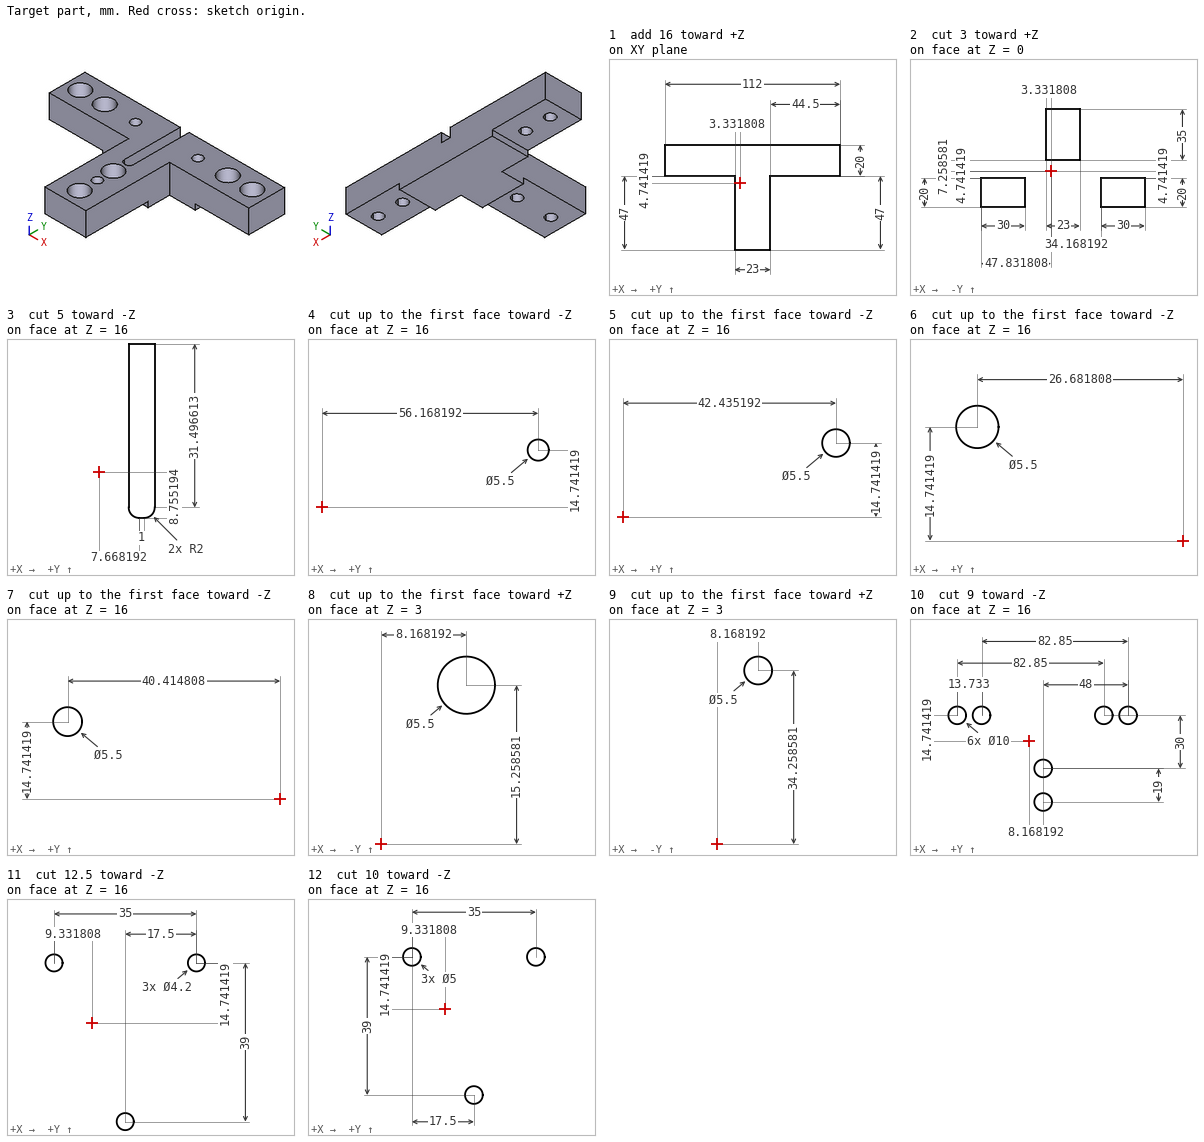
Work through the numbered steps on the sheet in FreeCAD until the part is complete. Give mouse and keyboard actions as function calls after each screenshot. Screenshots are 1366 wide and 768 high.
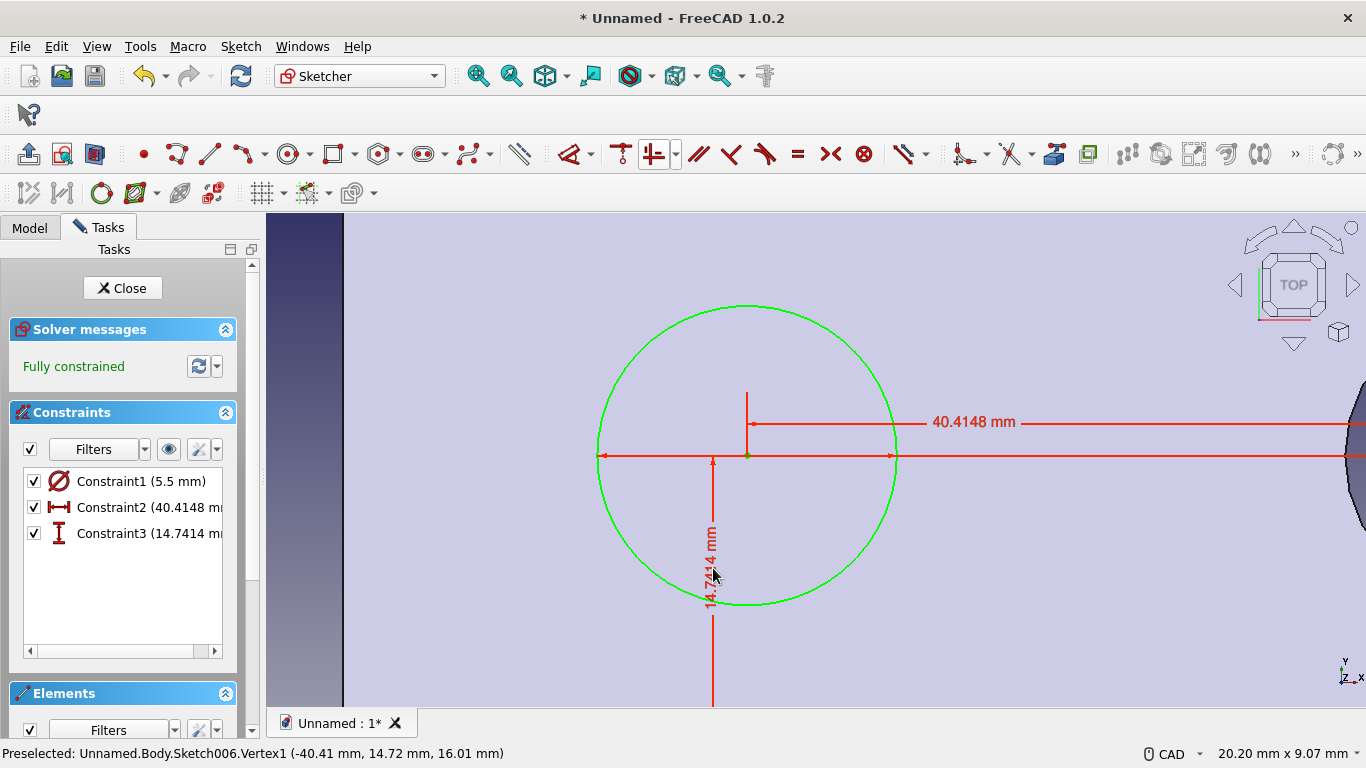
click(123, 288)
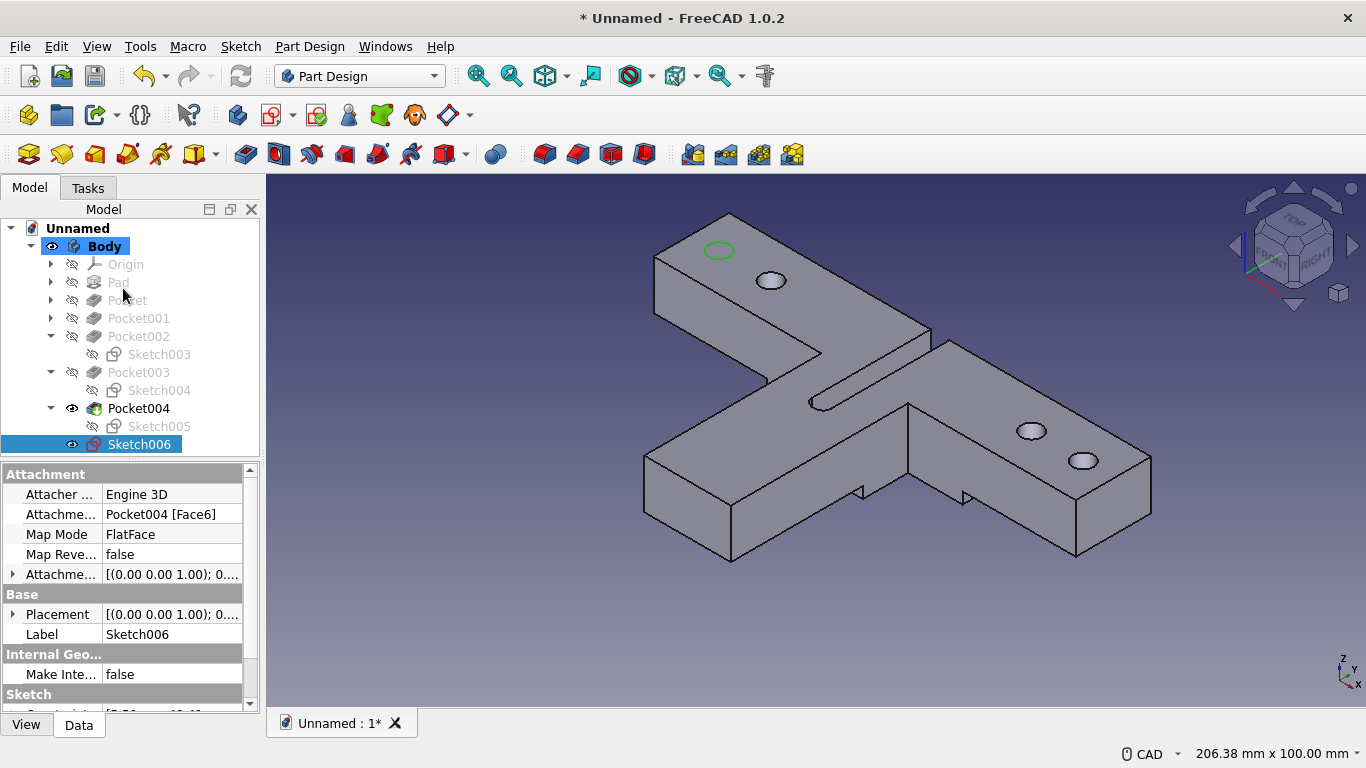
click(246, 154)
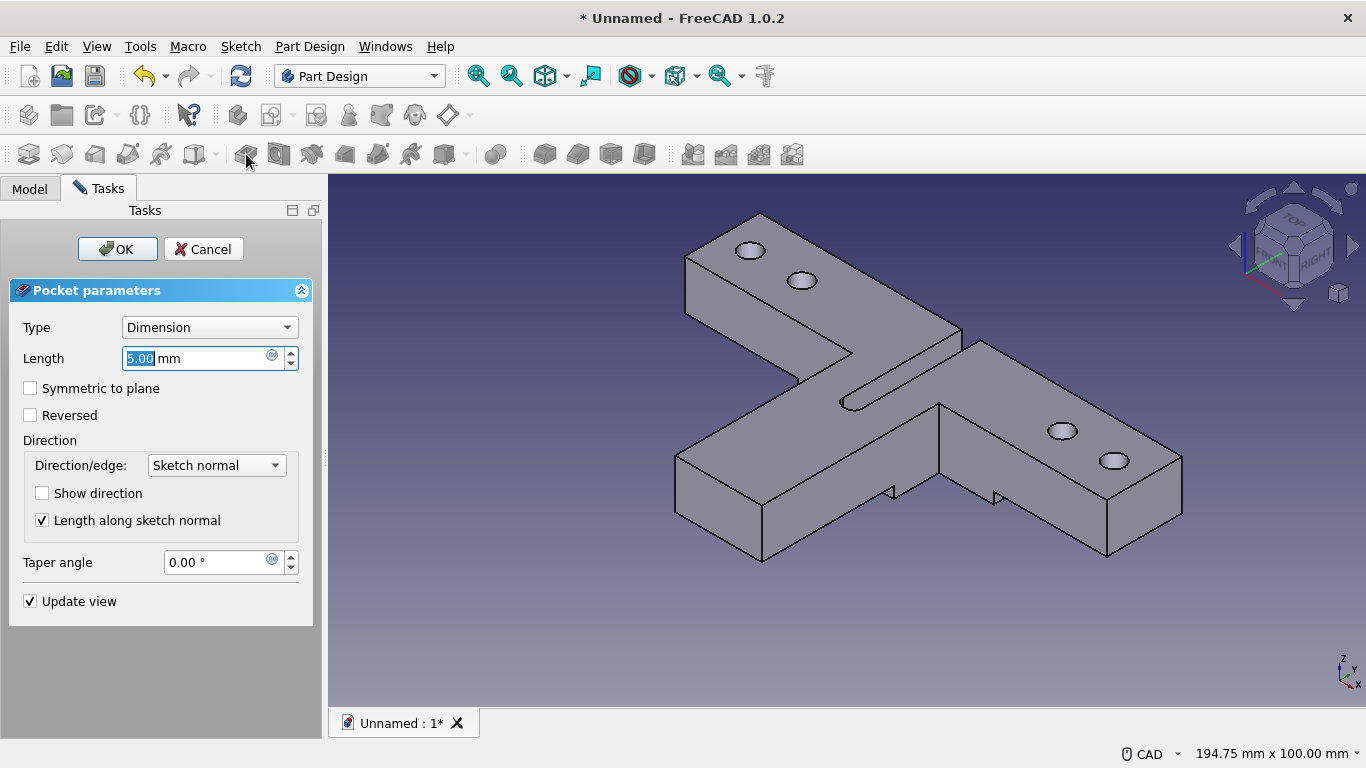
click(210, 328)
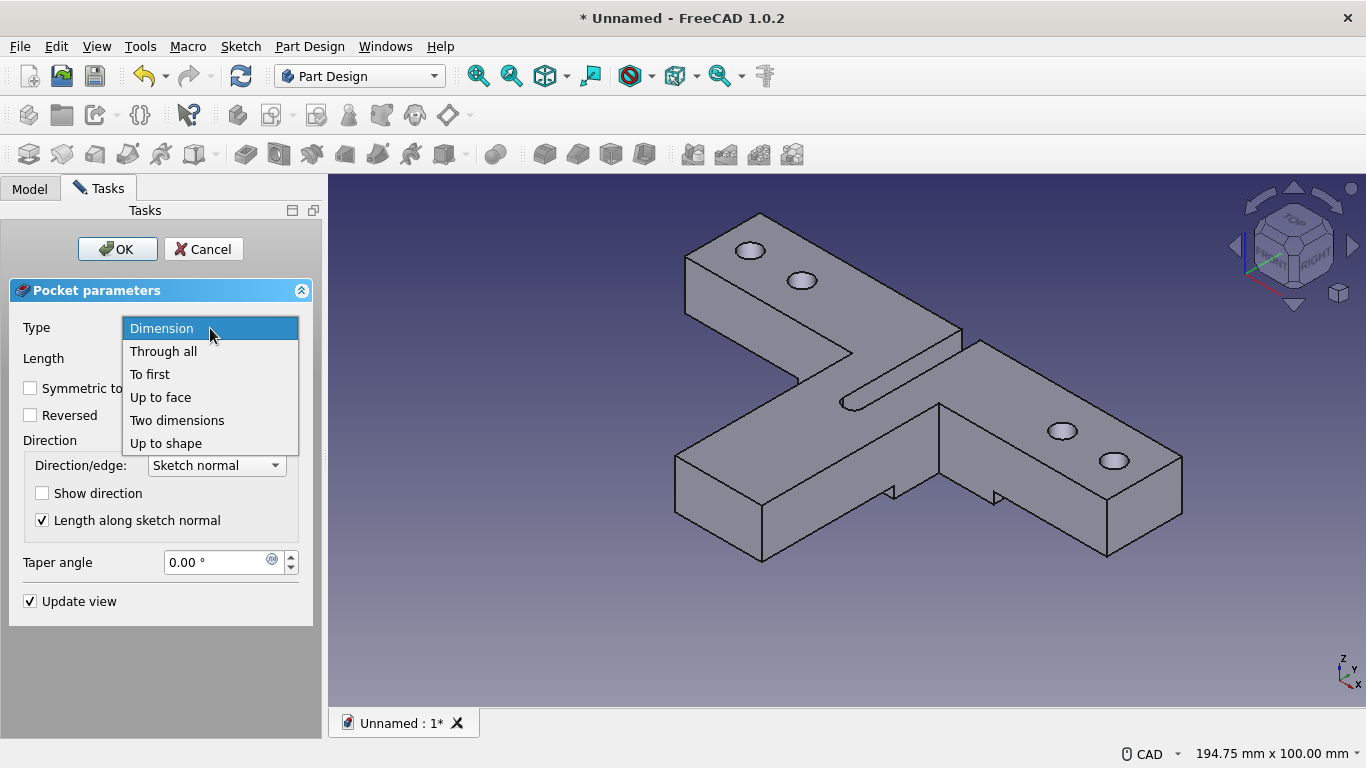
click(208, 374)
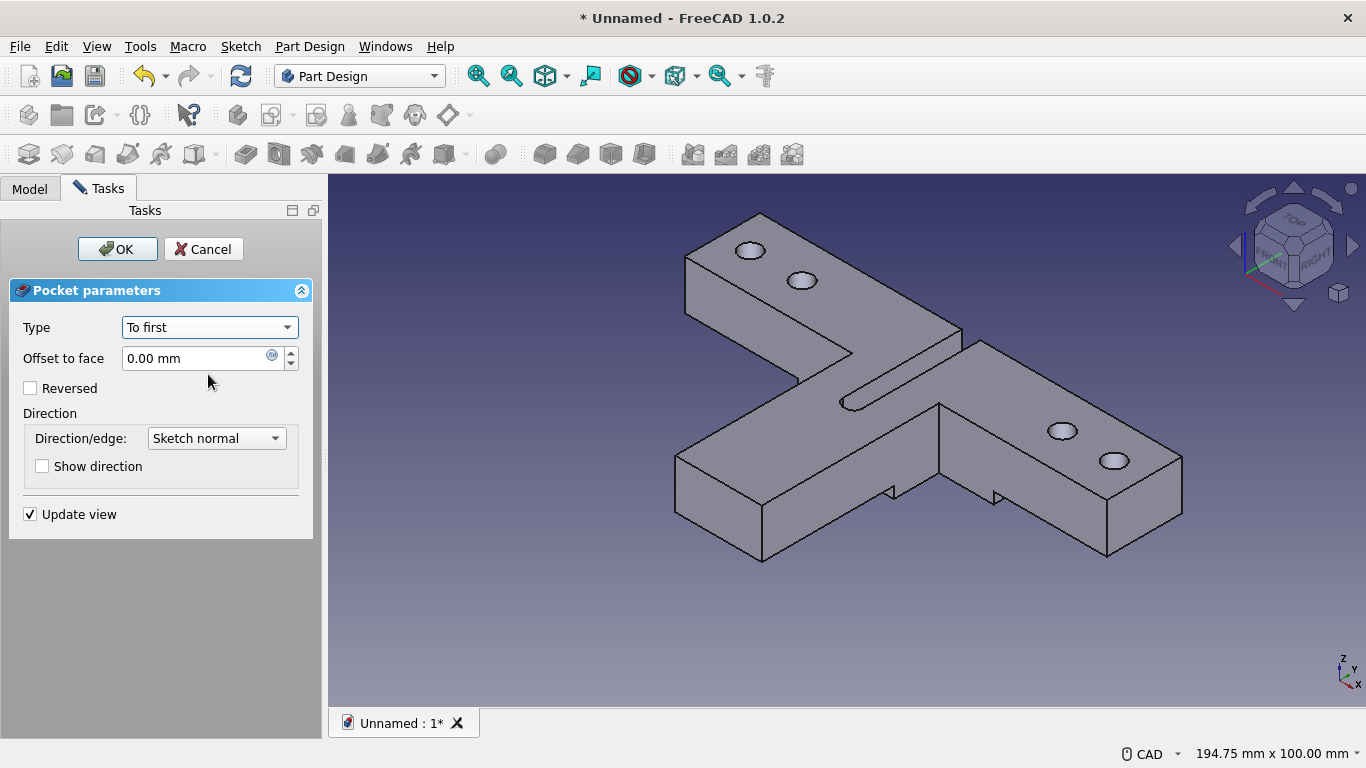
click(118, 249)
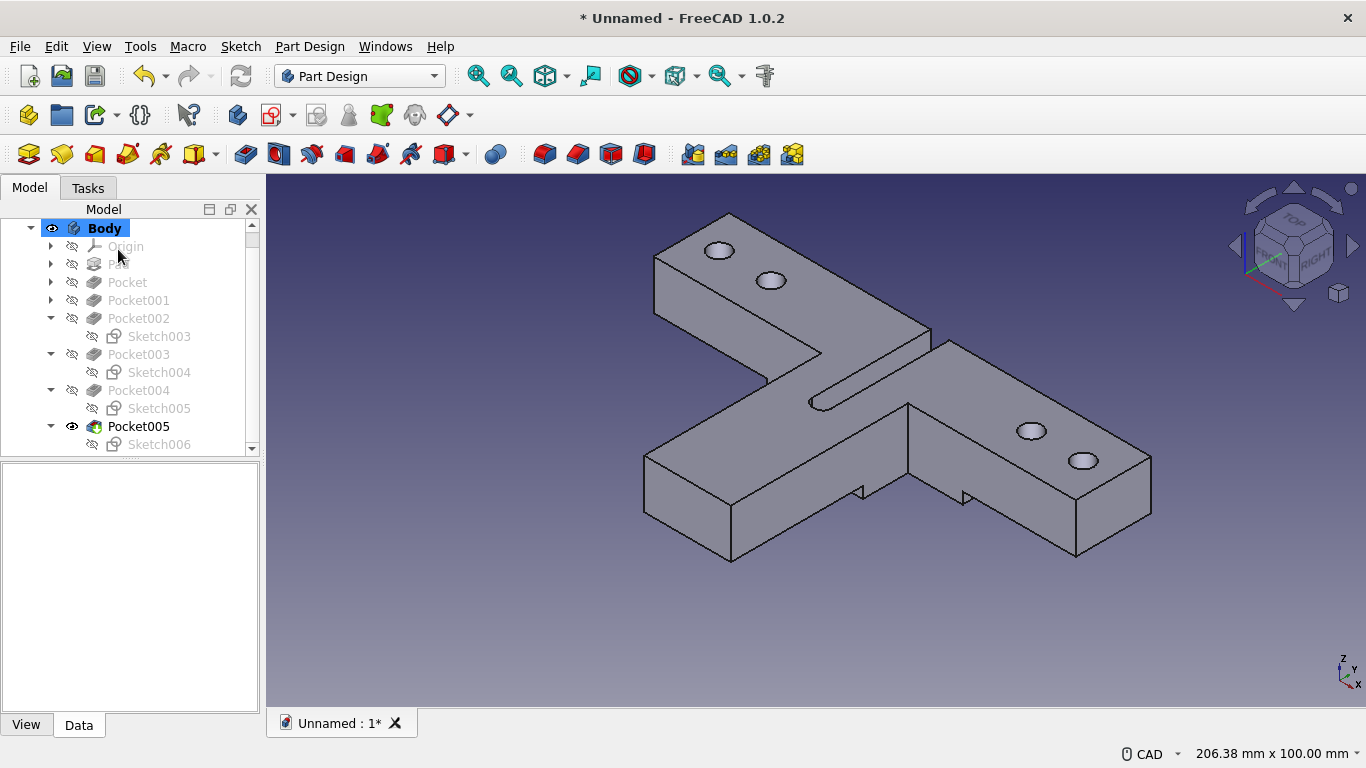
key(5)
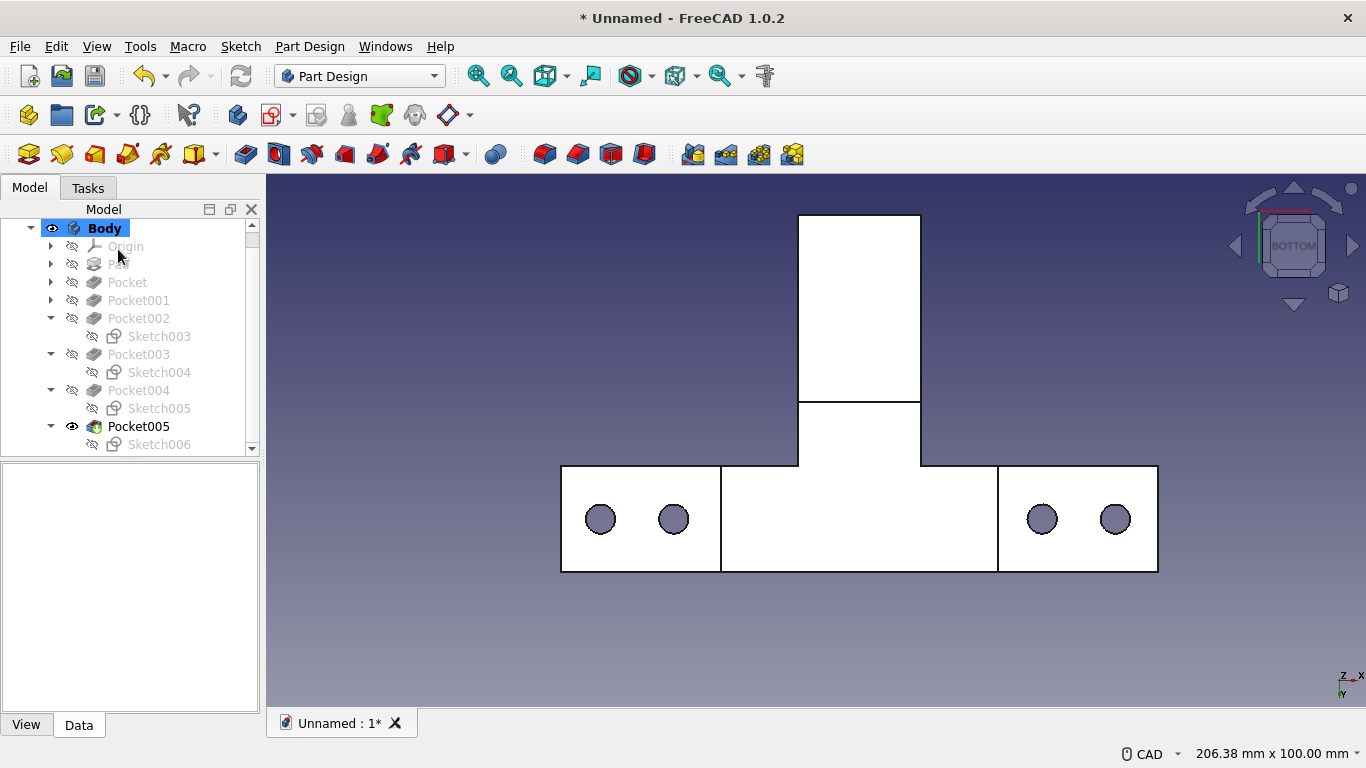
click(860, 334)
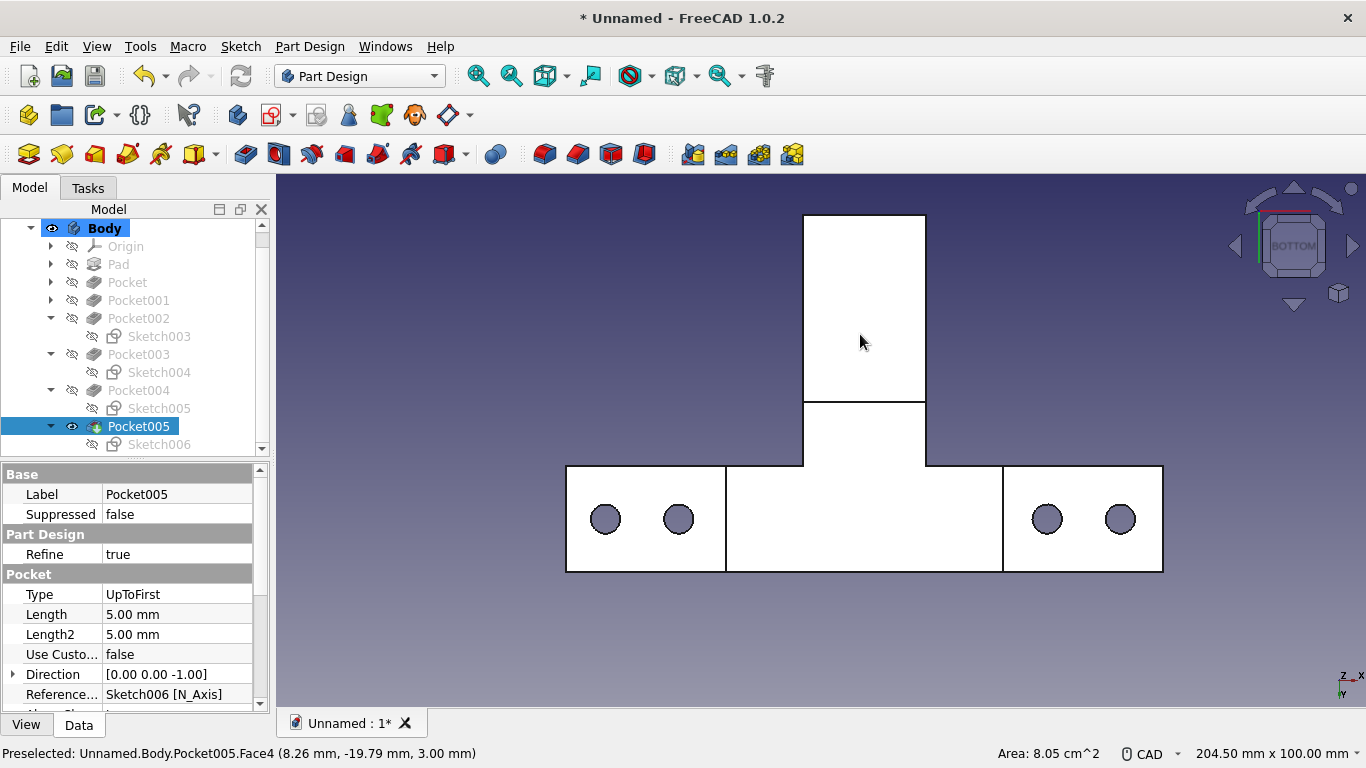
click(270, 116)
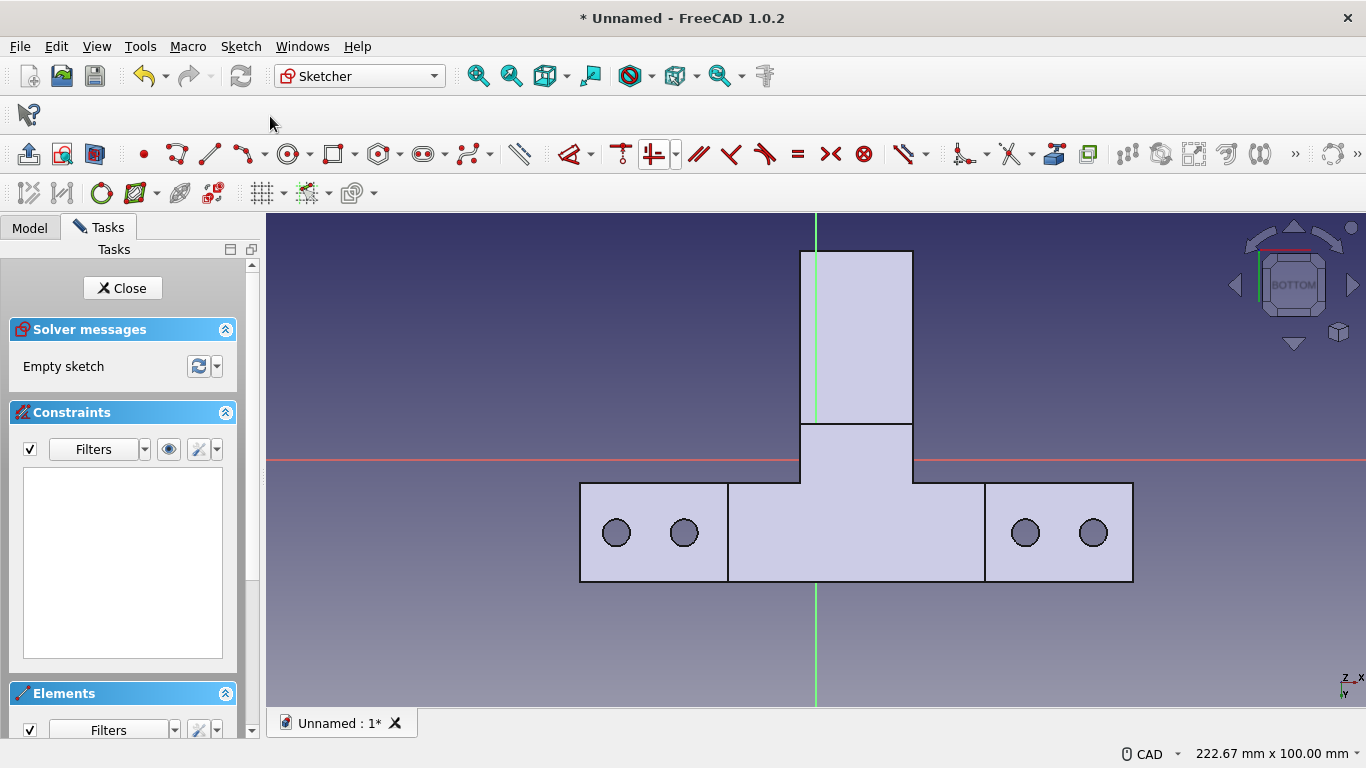
click(95, 154)